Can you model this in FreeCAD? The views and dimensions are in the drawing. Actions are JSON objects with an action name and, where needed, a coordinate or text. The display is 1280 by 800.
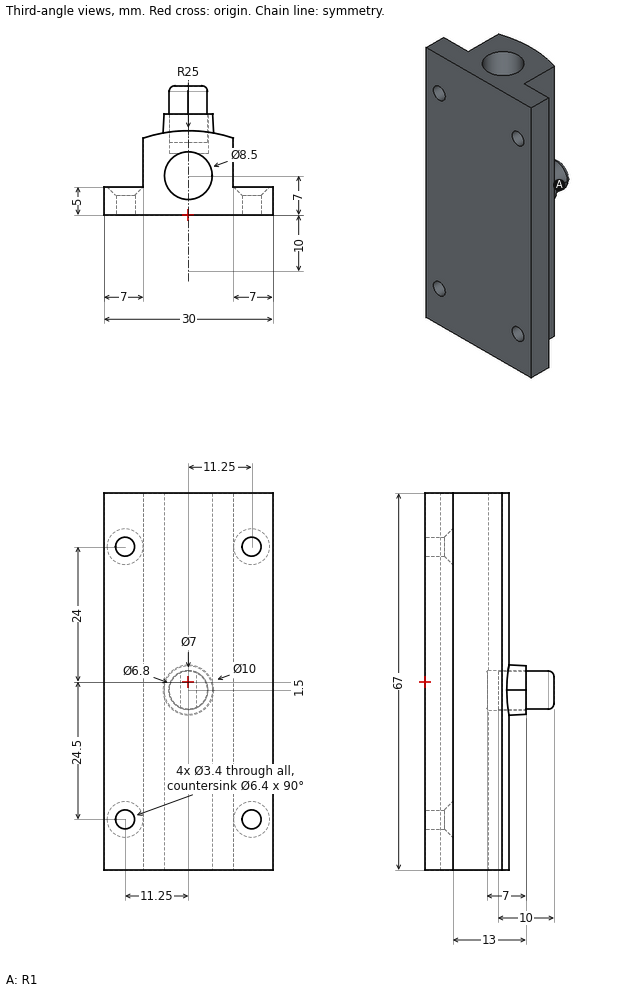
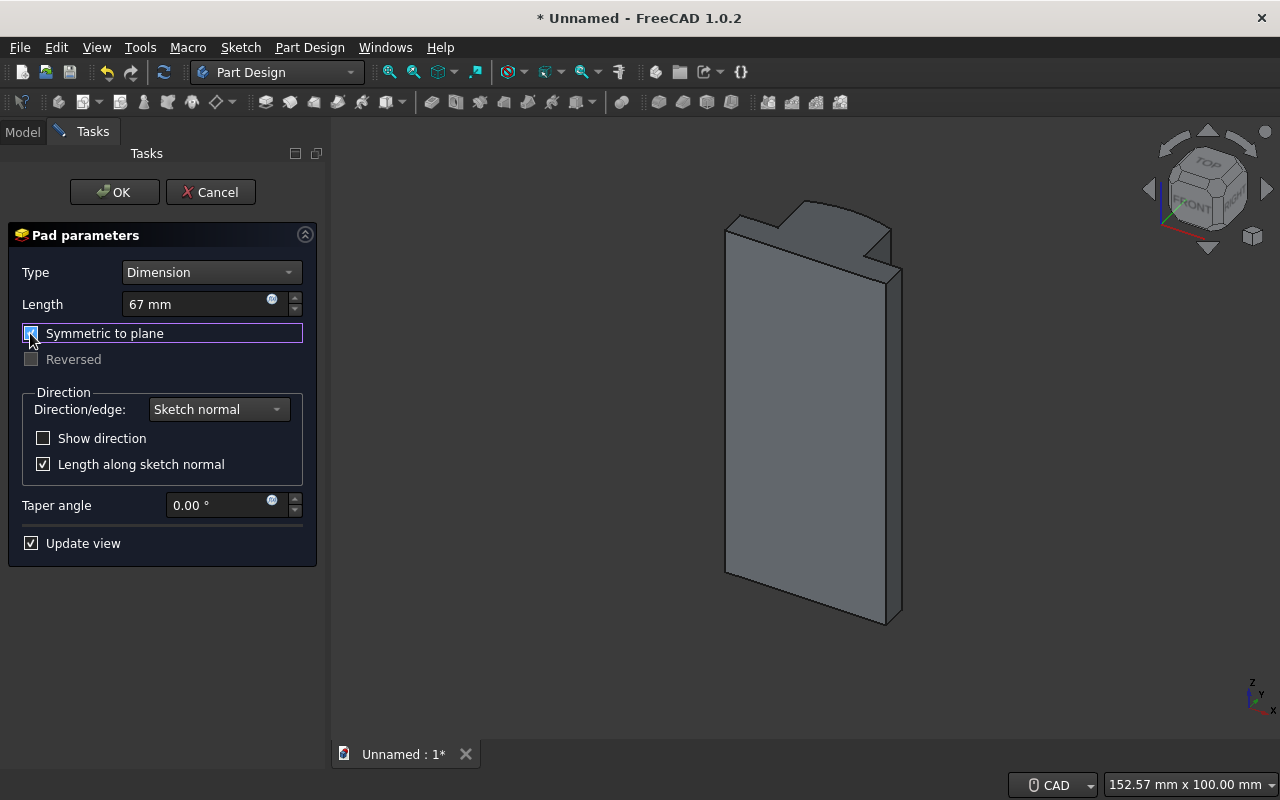
{"action": "left_click", "coordinate": [115, 192]}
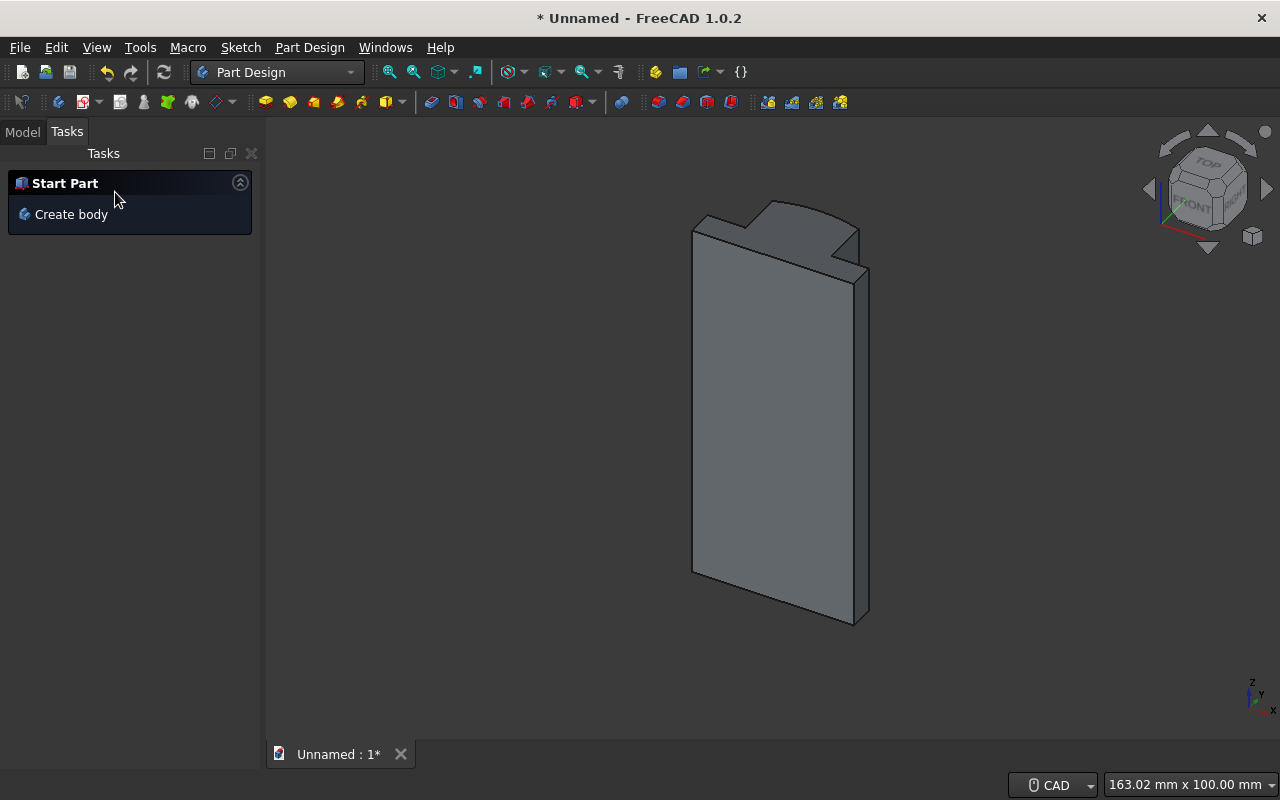
{"action": "key", "text": "4"}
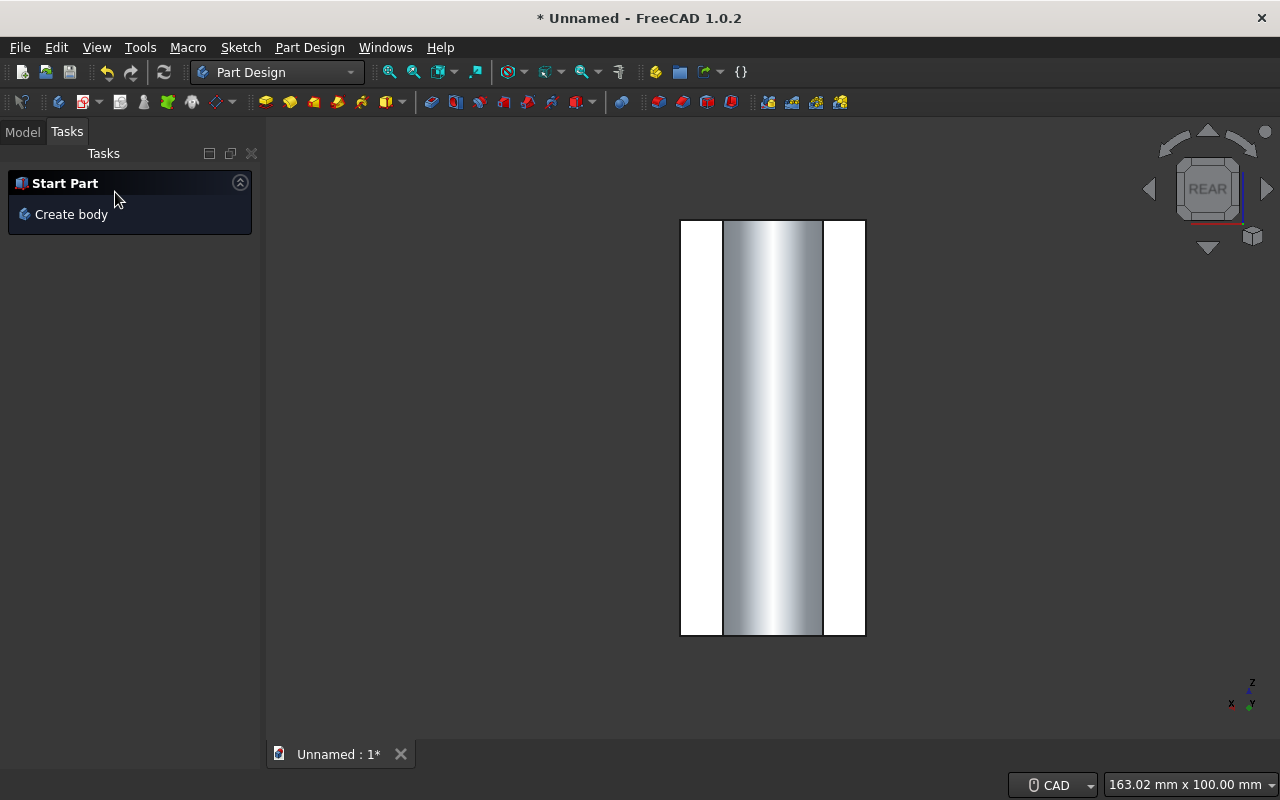
{"action": "left_click", "coordinate": [701, 248]}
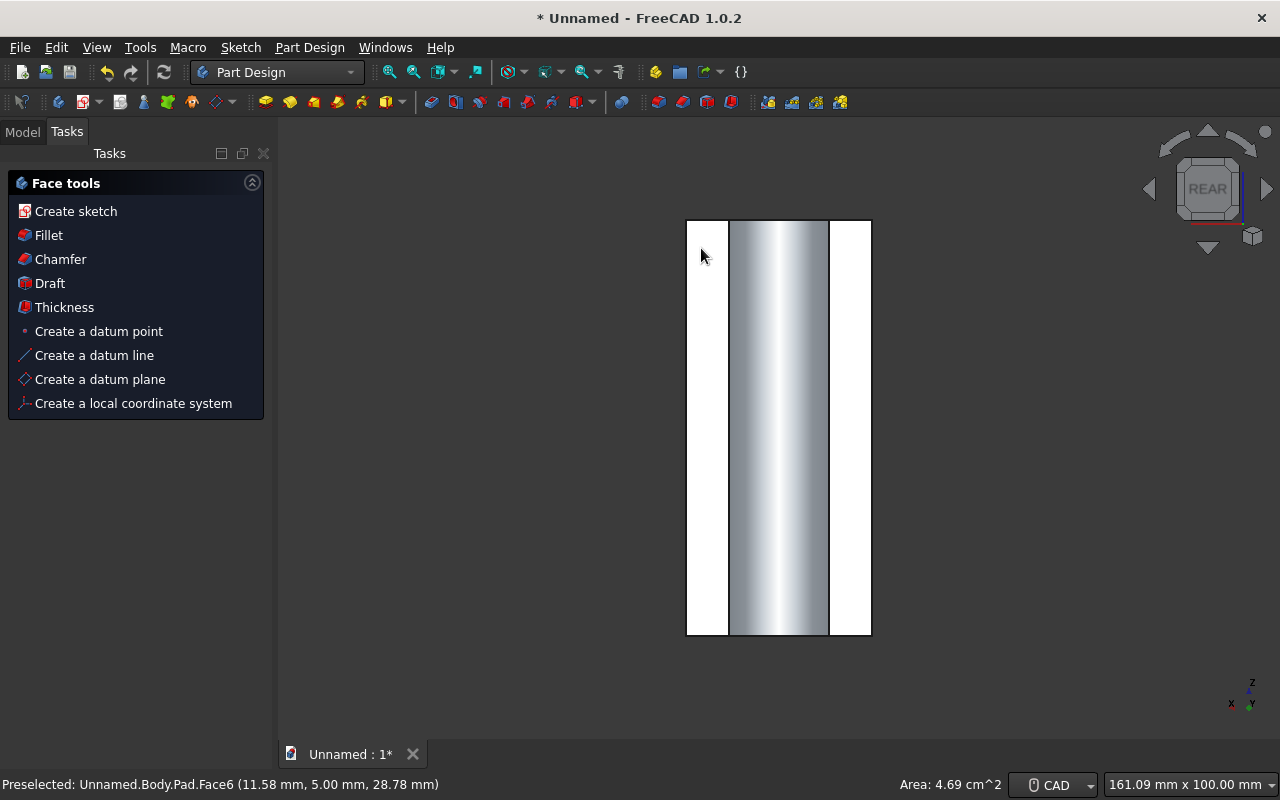
{"action": "left_click", "coordinate": [84, 102]}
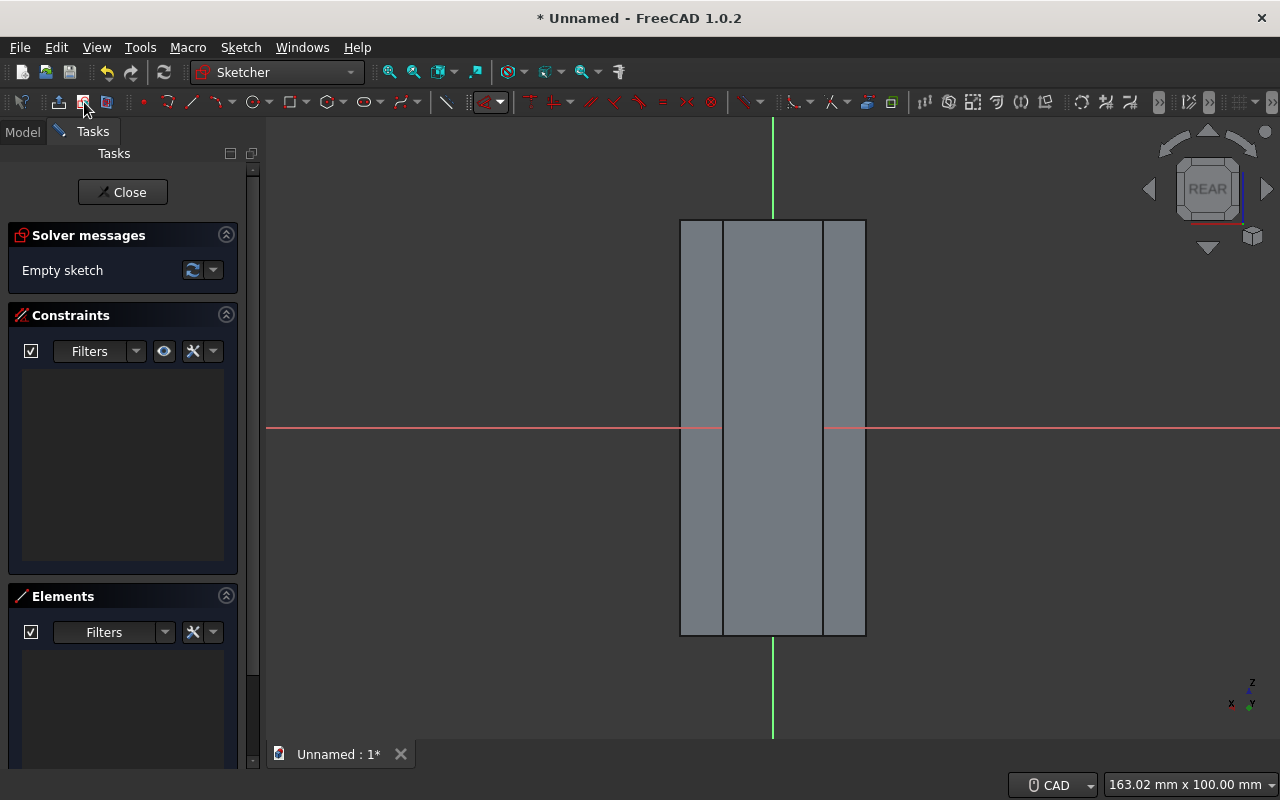
{"action": "key", "text": "q s"}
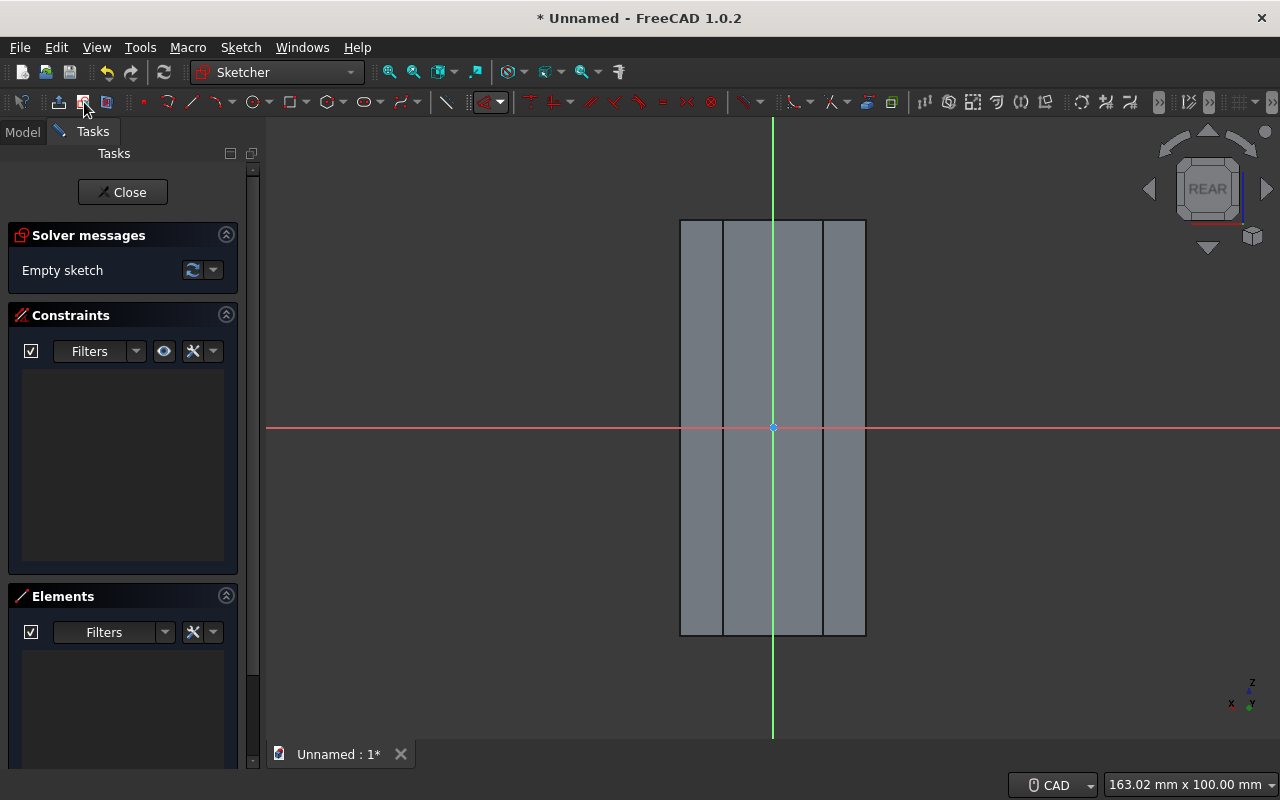
{"action": "key", "text": "g c"}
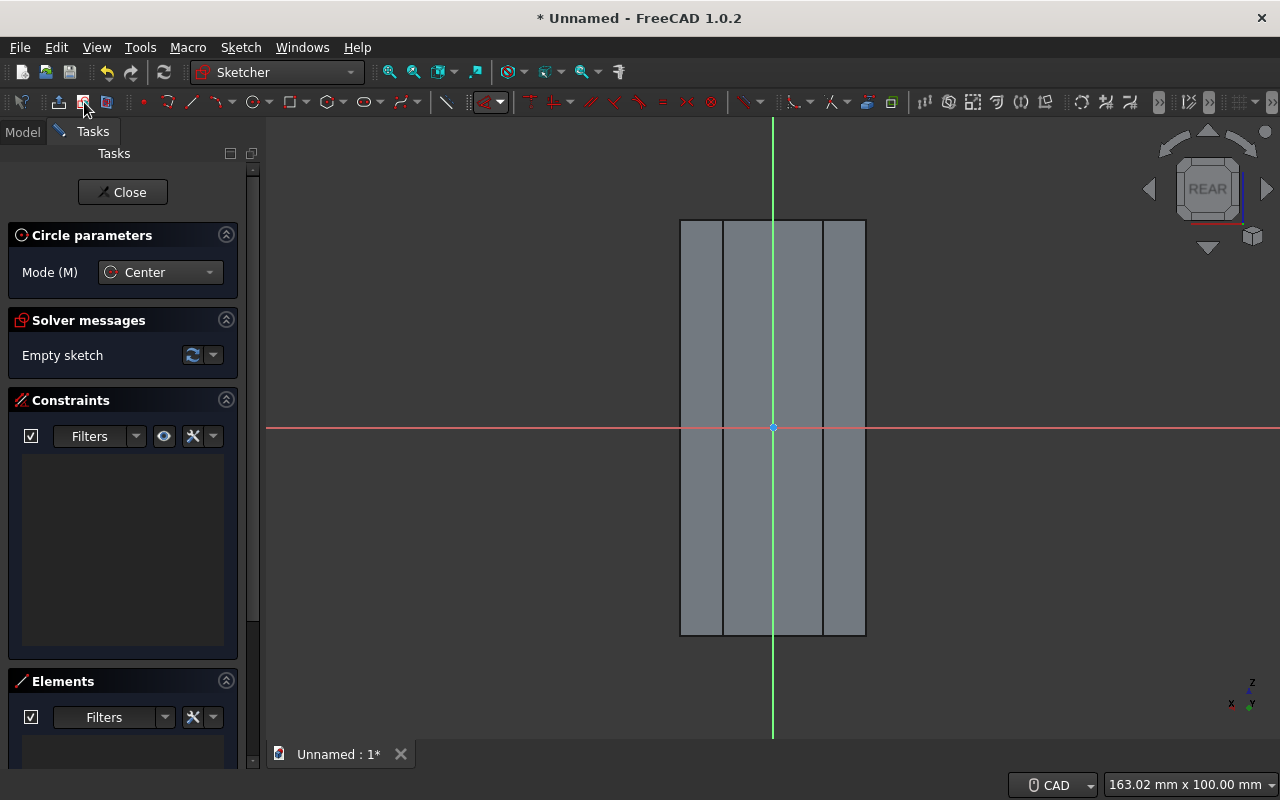
{"action": "scroll", "coordinate": [843, 580], "scroll_direction": "up", "scroll_amount": 4}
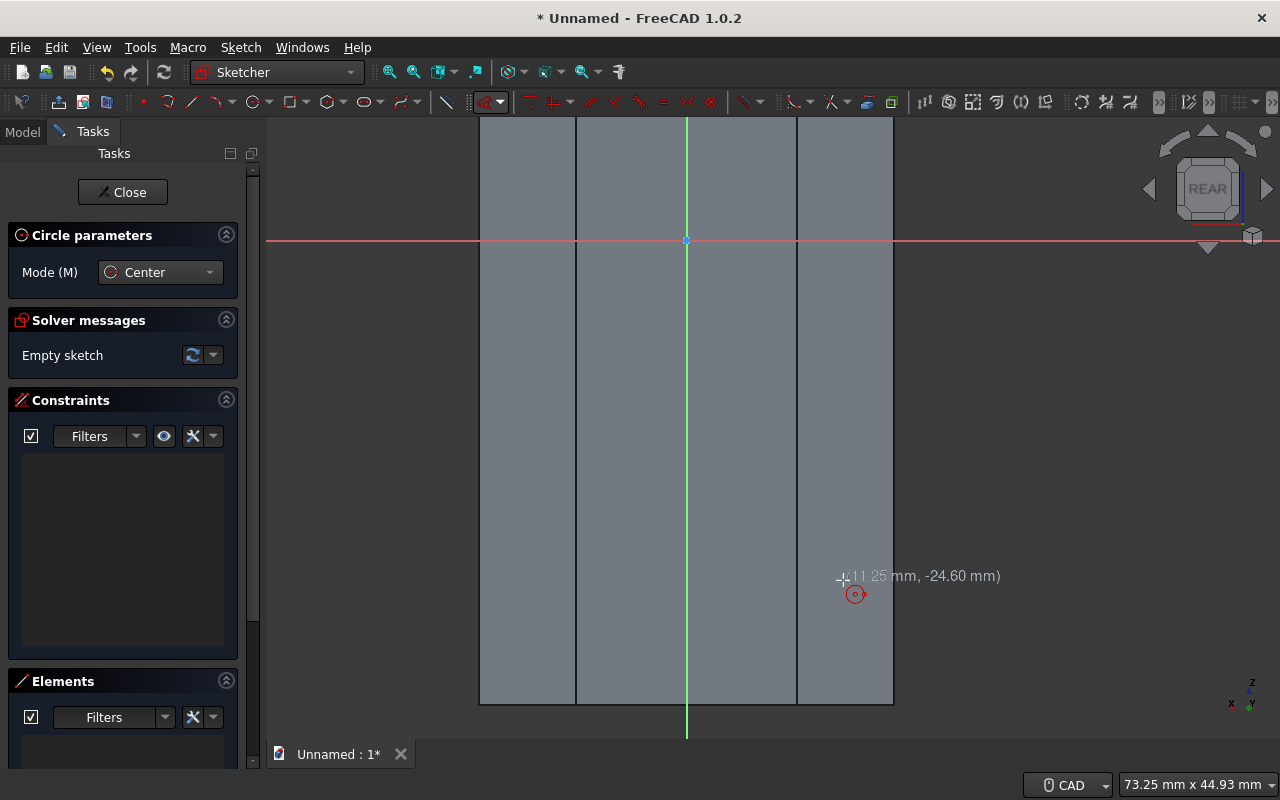
{"action": "left_click", "coordinate": [842, 580]}
{"action": "left_click", "coordinate": [859, 563]}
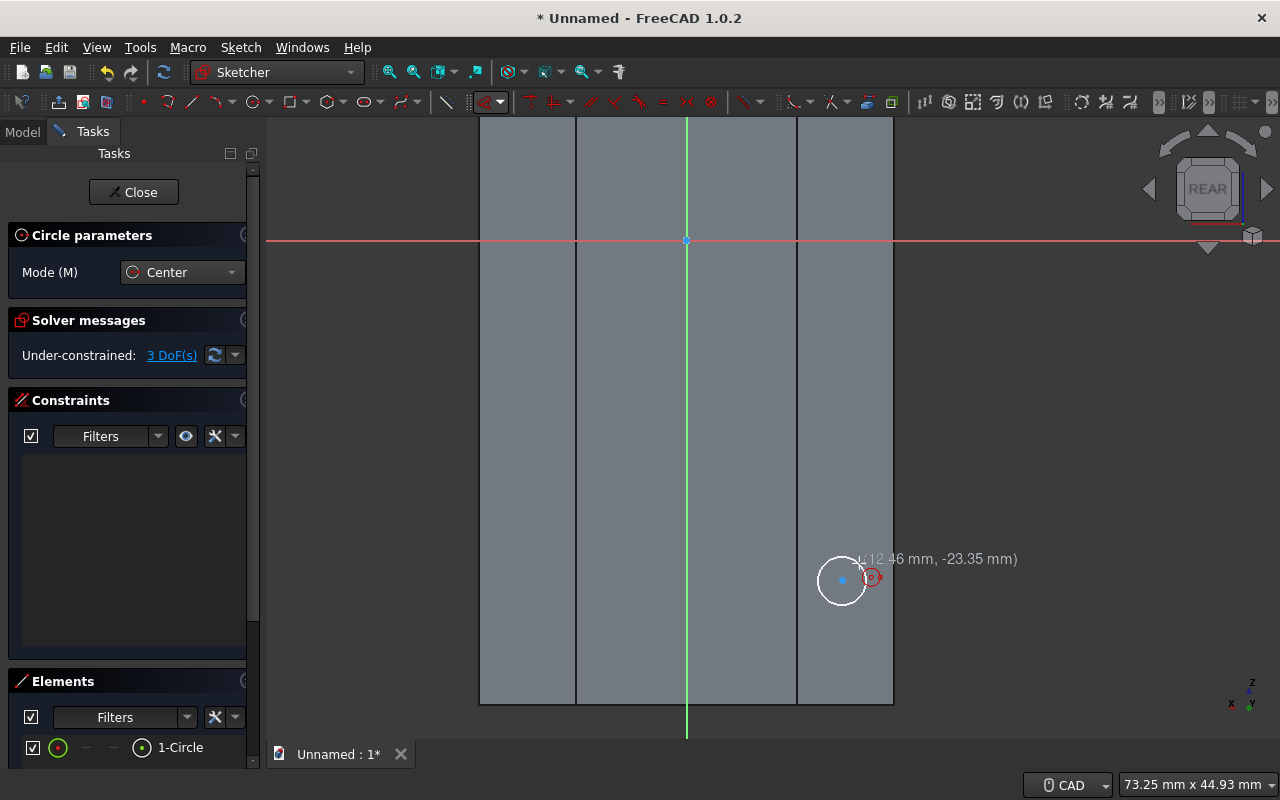
{"action": "scroll", "coordinate": [726, 651], "scroll_direction": "down", "scroll_amount": 3}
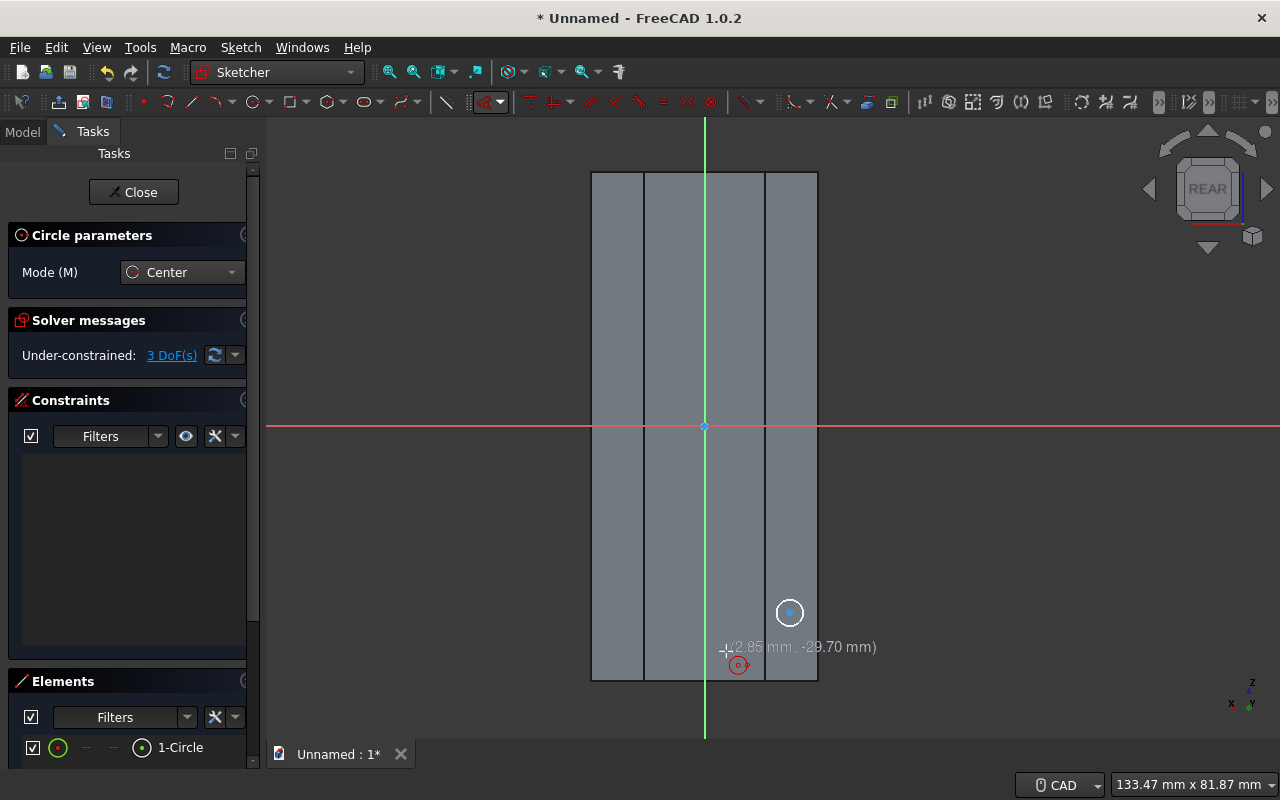
{"action": "scroll", "coordinate": [790, 244], "scroll_direction": "up", "scroll_amount": 3}